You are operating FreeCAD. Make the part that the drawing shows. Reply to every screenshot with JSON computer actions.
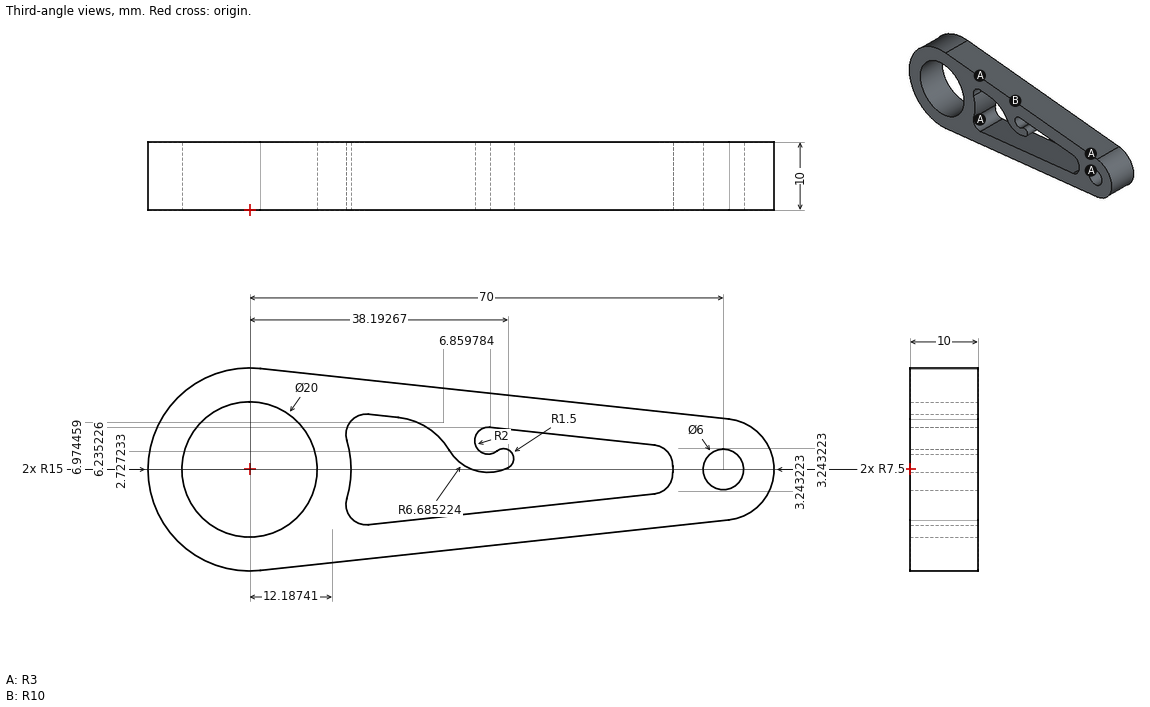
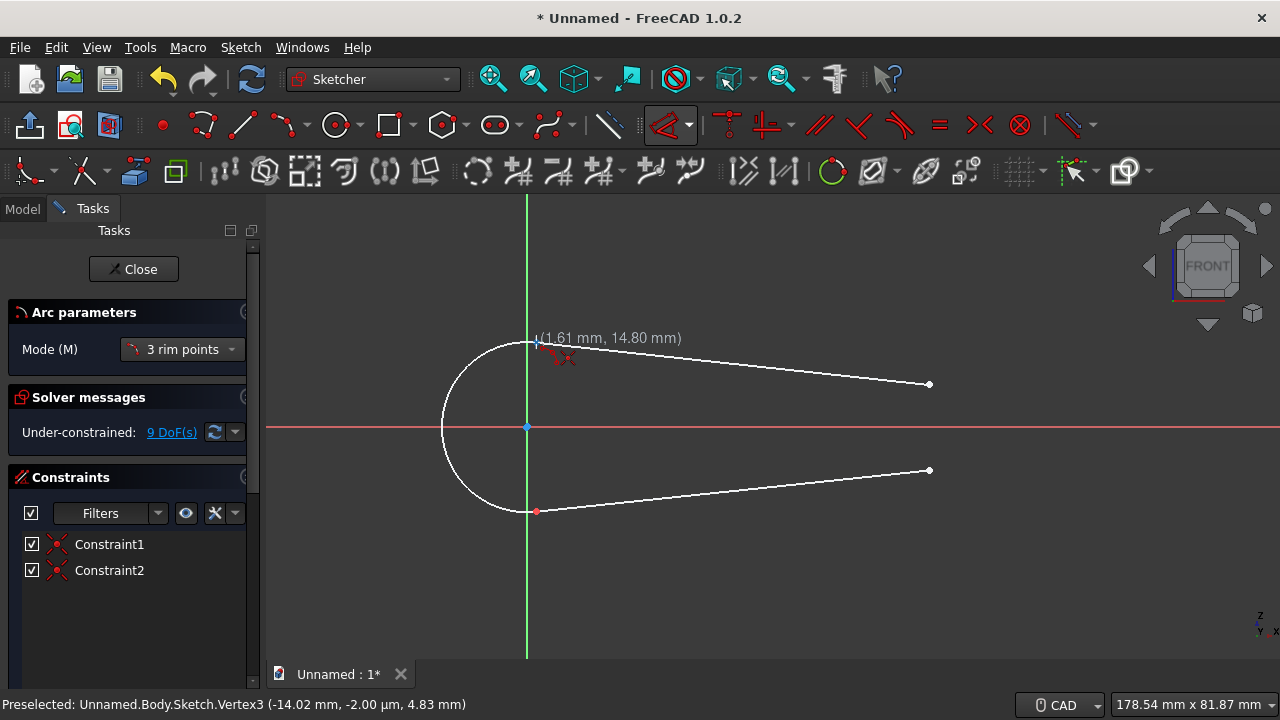
{"action": "left_click", "coordinate": [929, 385]}
{"action": "left_click", "coordinate": [929, 470]}
{"action": "left_click", "coordinate": [960, 450]}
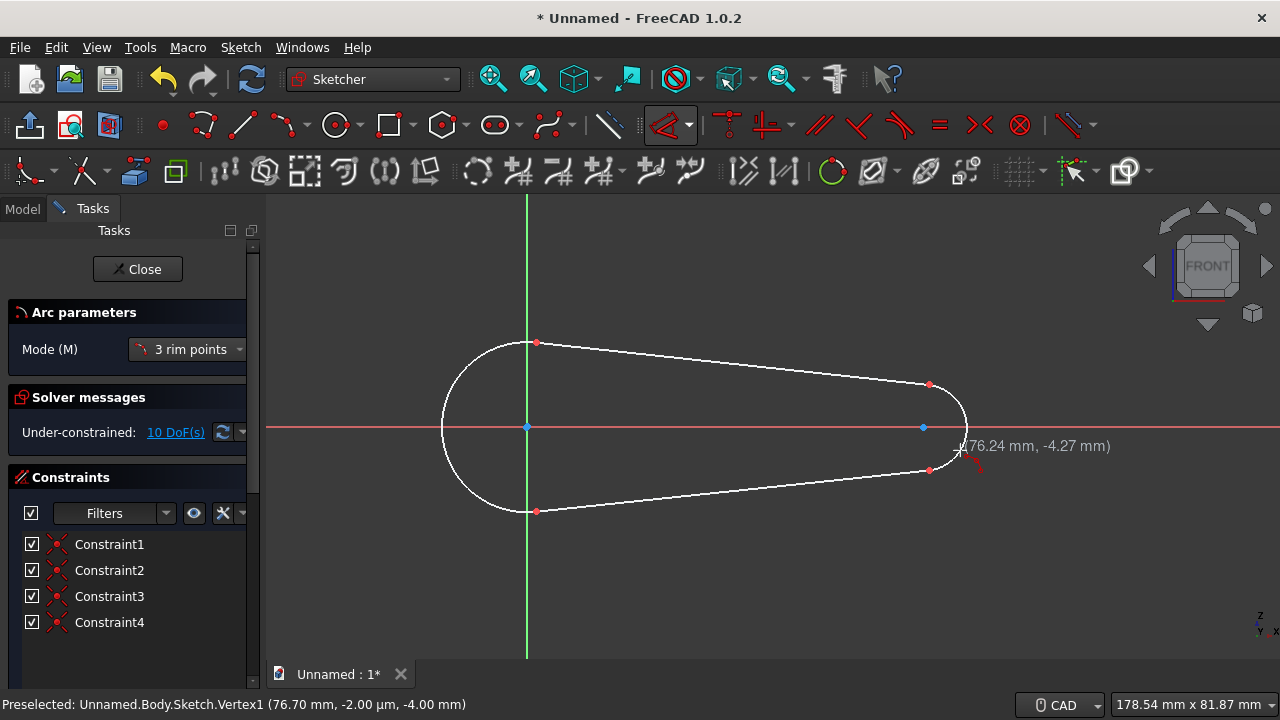
{"action": "key", "text": "g l"}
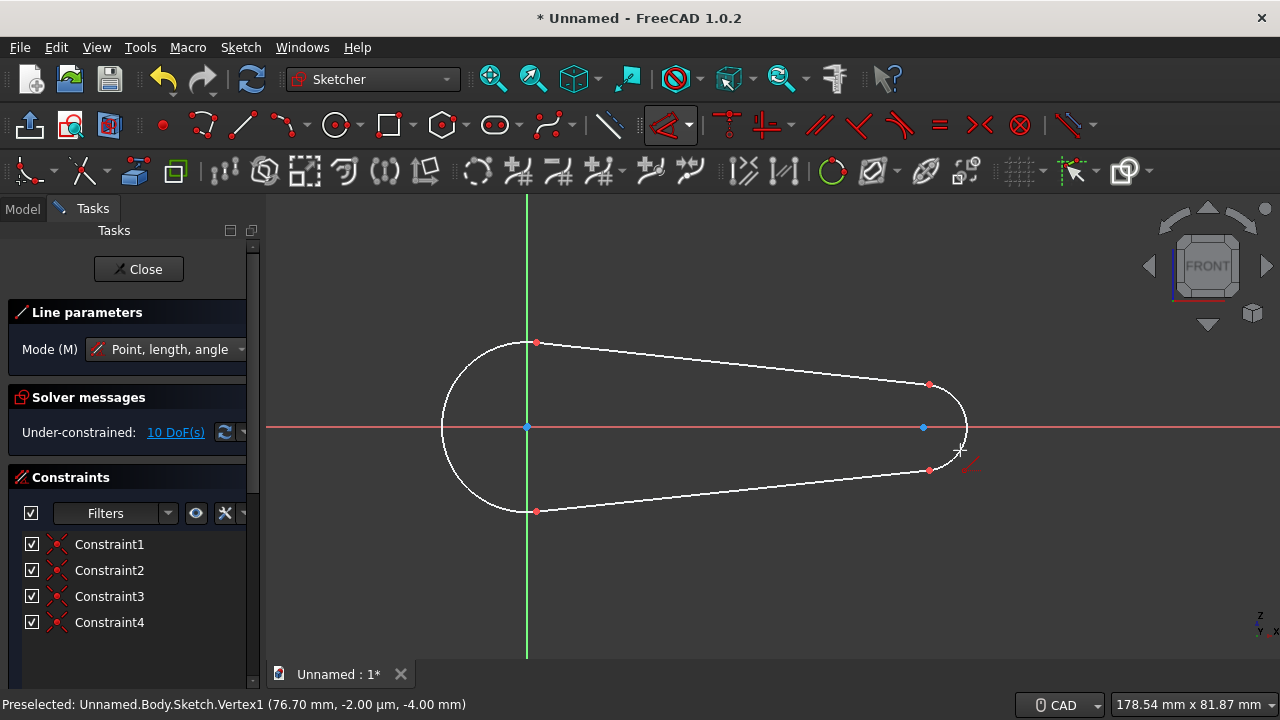
{"action": "left_click", "coordinate": [596, 476]}
{"action": "left_click", "coordinate": [886, 445]}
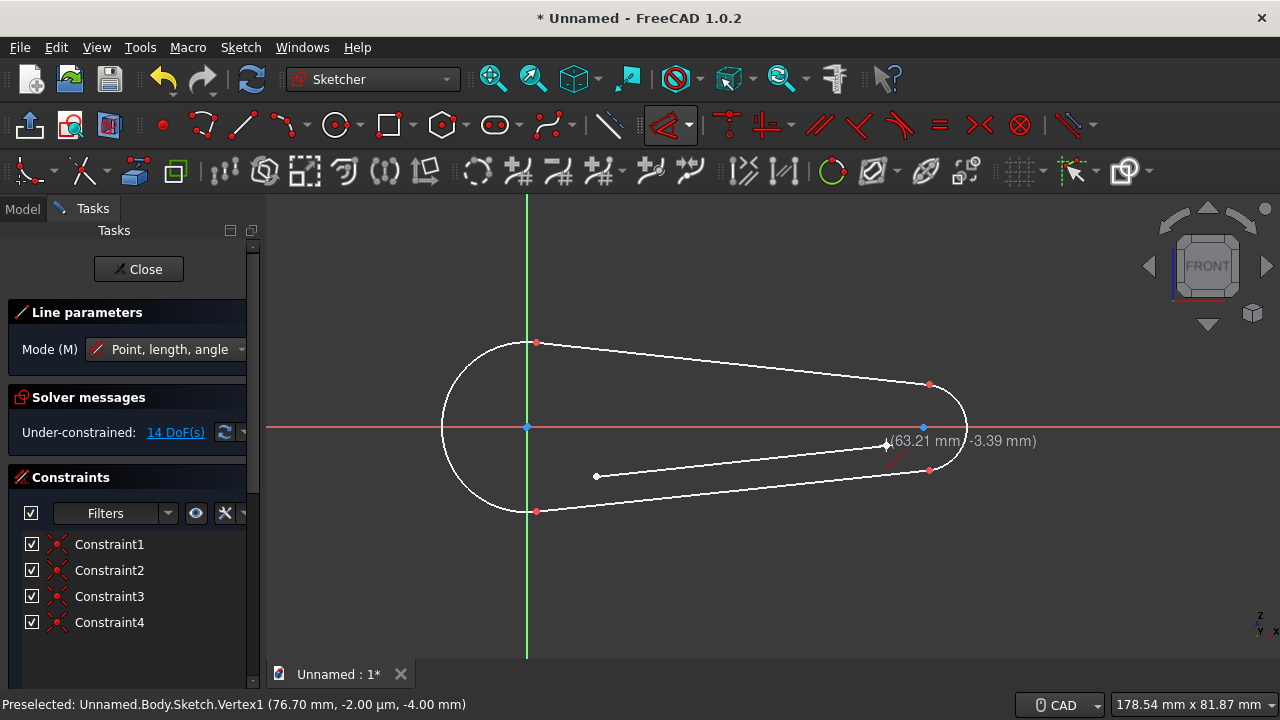
{"action": "left_click", "coordinate": [886, 408]}
{"action": "left_click", "coordinate": [596, 377]}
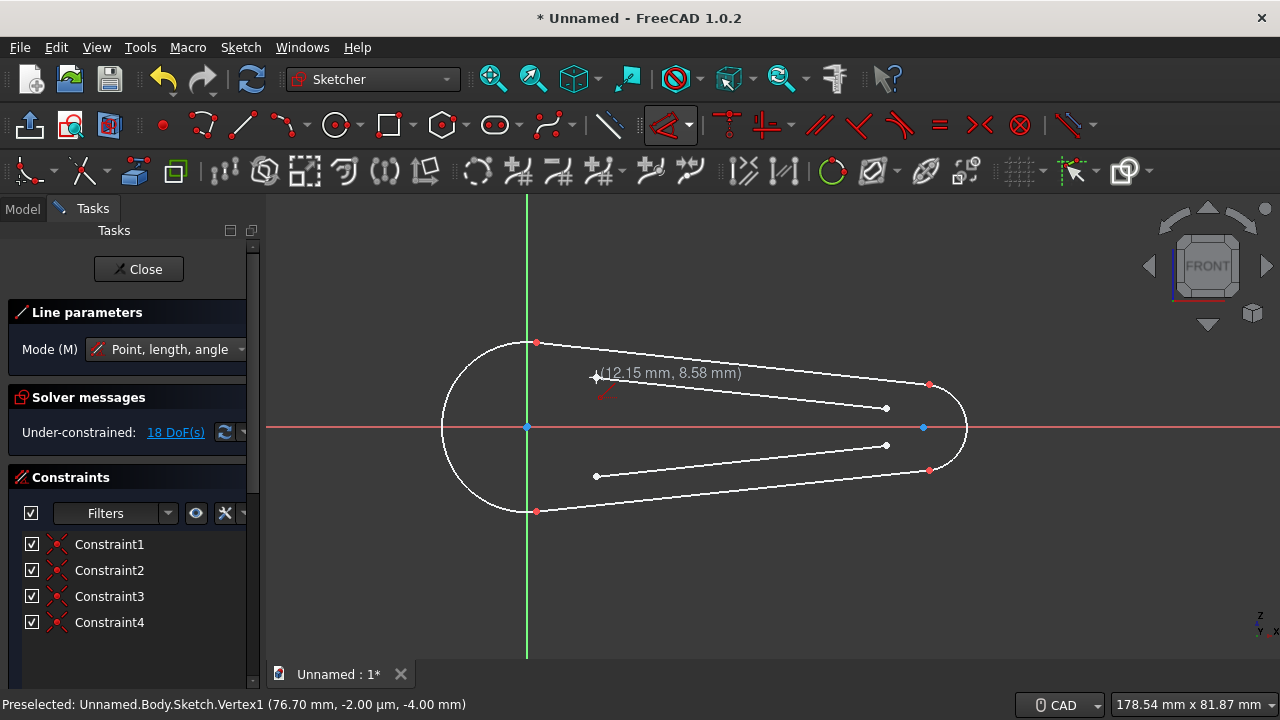
{"action": "left_click", "coordinate": [284, 126]}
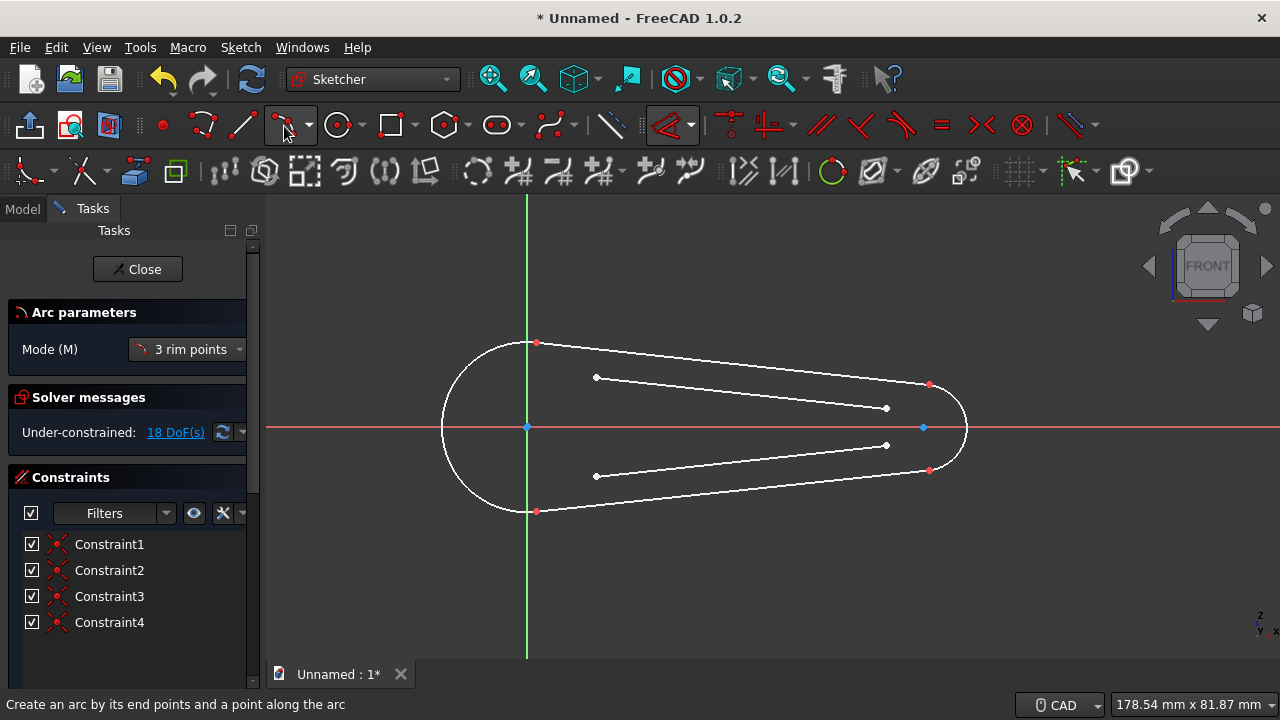
{"action": "left_click", "coordinate": [886, 446]}
{"action": "left_click", "coordinate": [886, 409]}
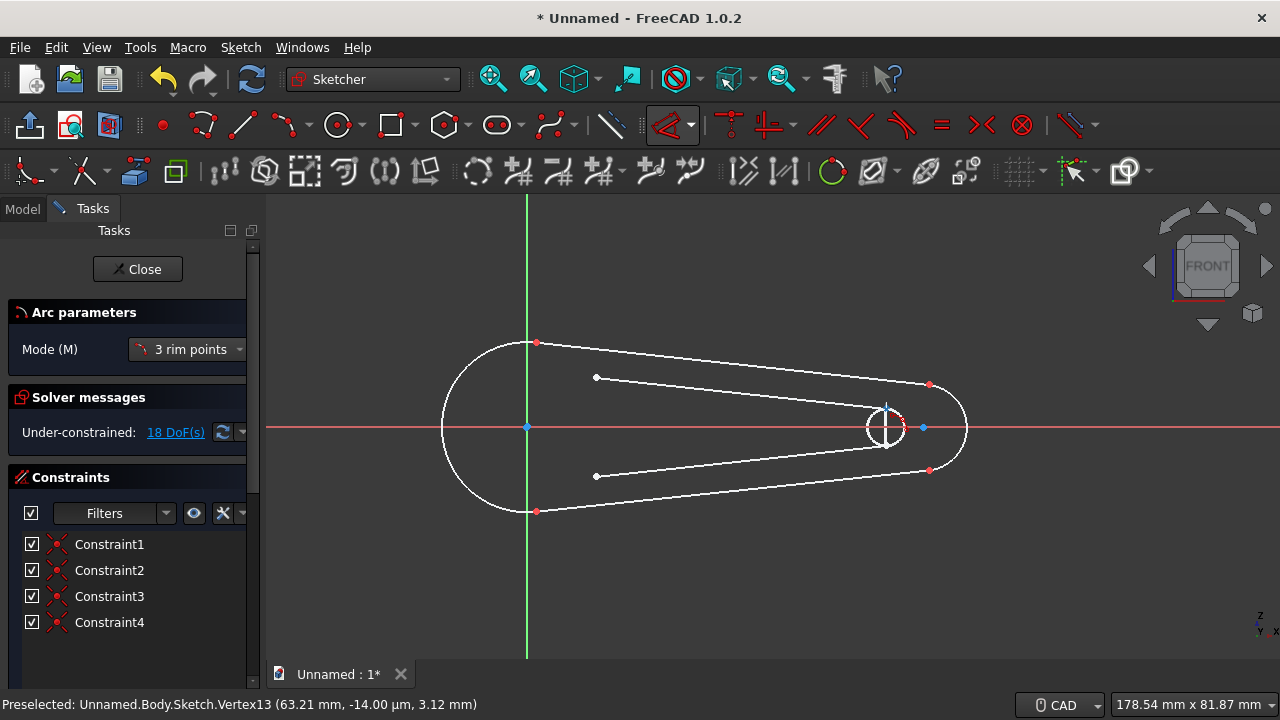
{"action": "scroll", "coordinate": [882, 423], "scroll_direction": "up", "scroll_amount": 8}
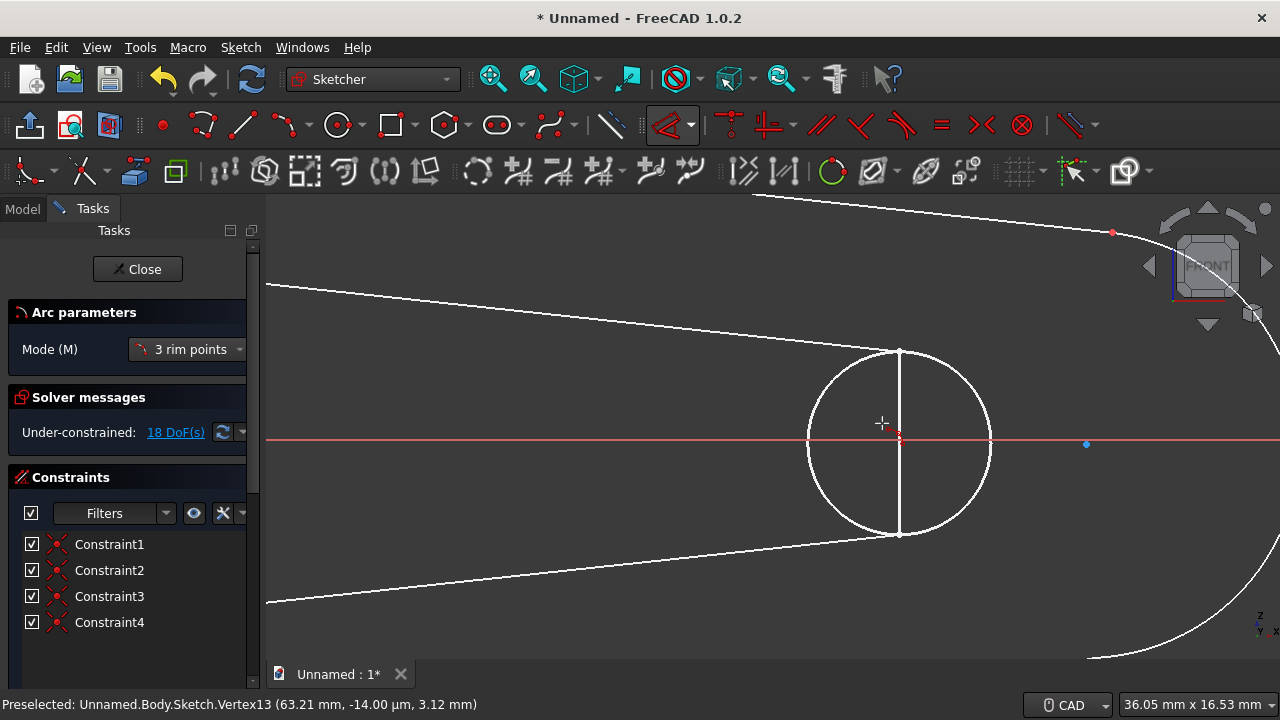
{"action": "left_click", "coordinate": [880, 421]}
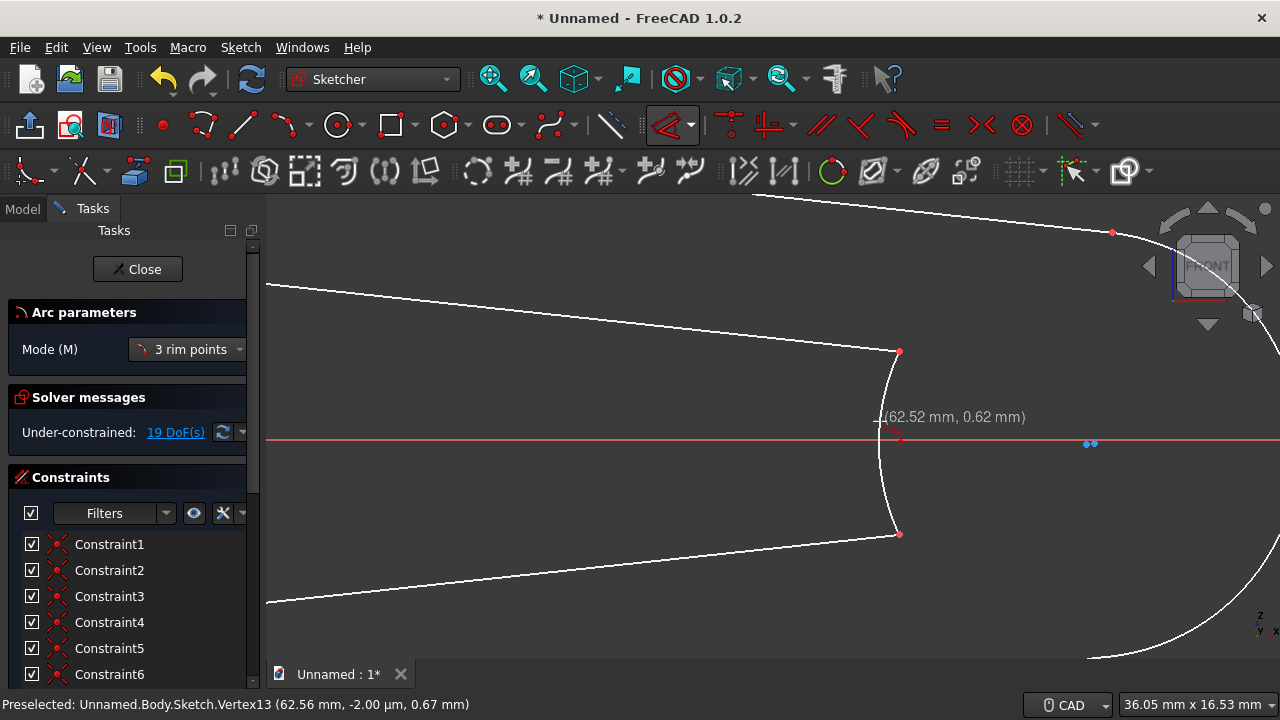
{"action": "scroll", "coordinate": [883, 423], "scroll_direction": "down", "scroll_amount": 8}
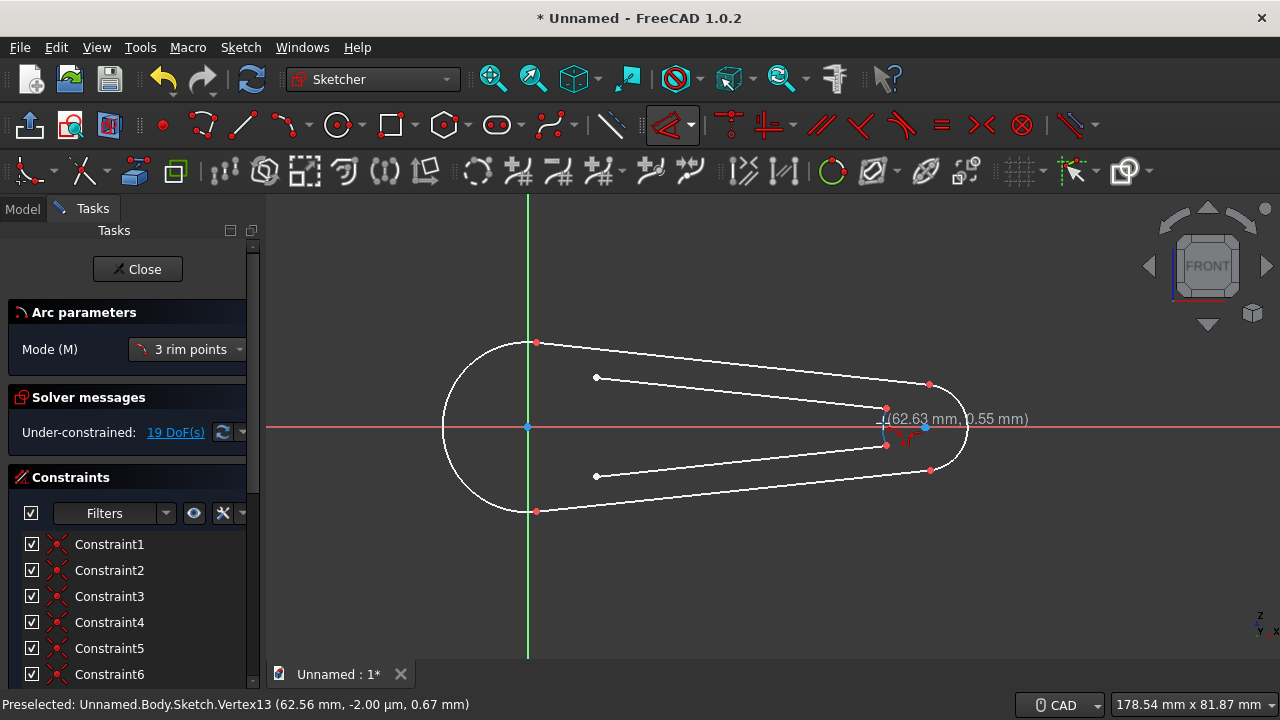
{"action": "left_click", "coordinate": [597, 378]}
{"action": "left_click", "coordinate": [597, 477]}
{"action": "left_click", "coordinate": [610, 448]}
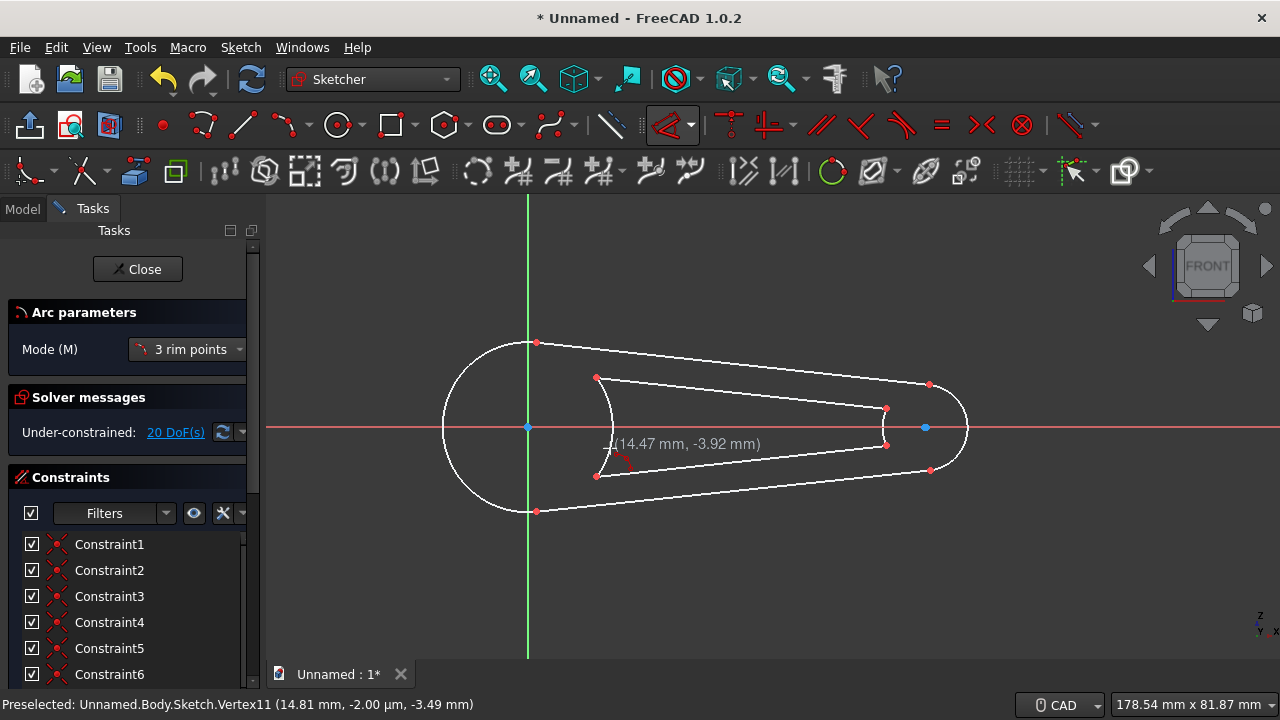
{"action": "key", "text": "g c"}